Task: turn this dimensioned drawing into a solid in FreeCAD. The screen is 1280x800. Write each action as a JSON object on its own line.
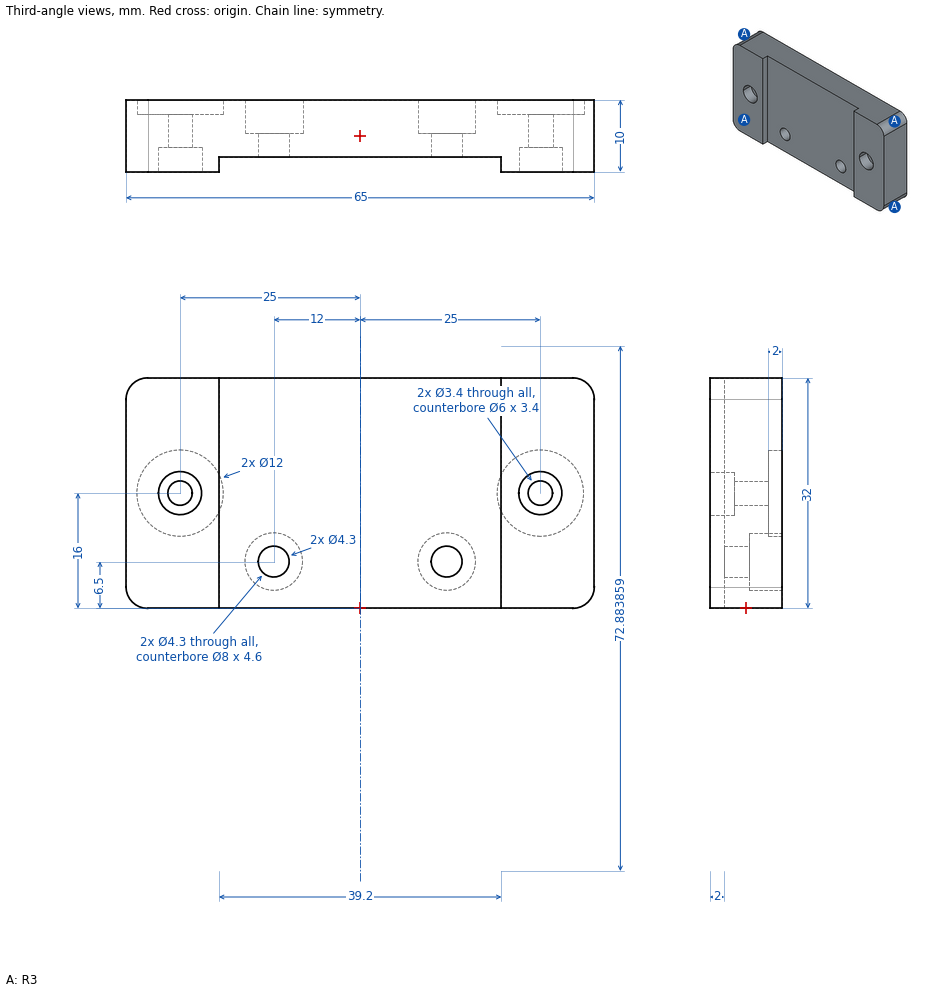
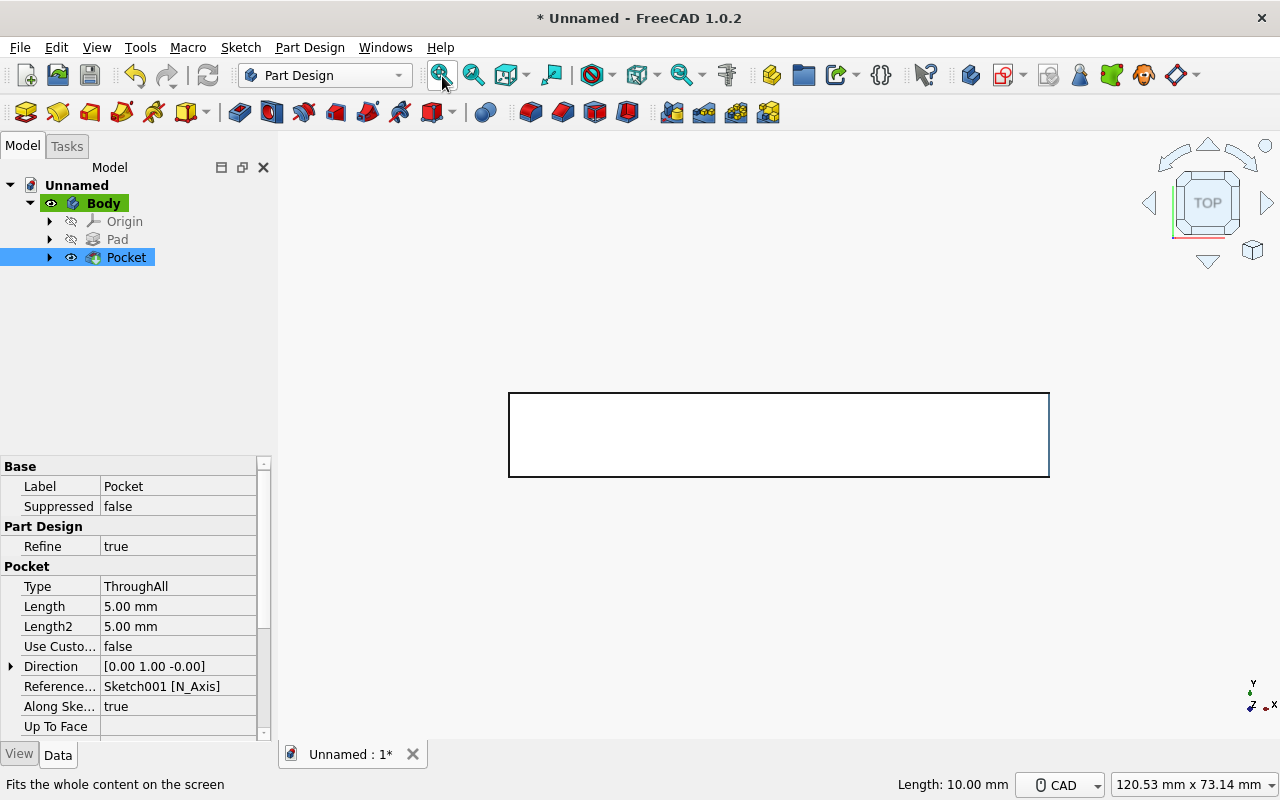
{"action": "left_click", "coordinate": [509, 434], "text": "ctrl"}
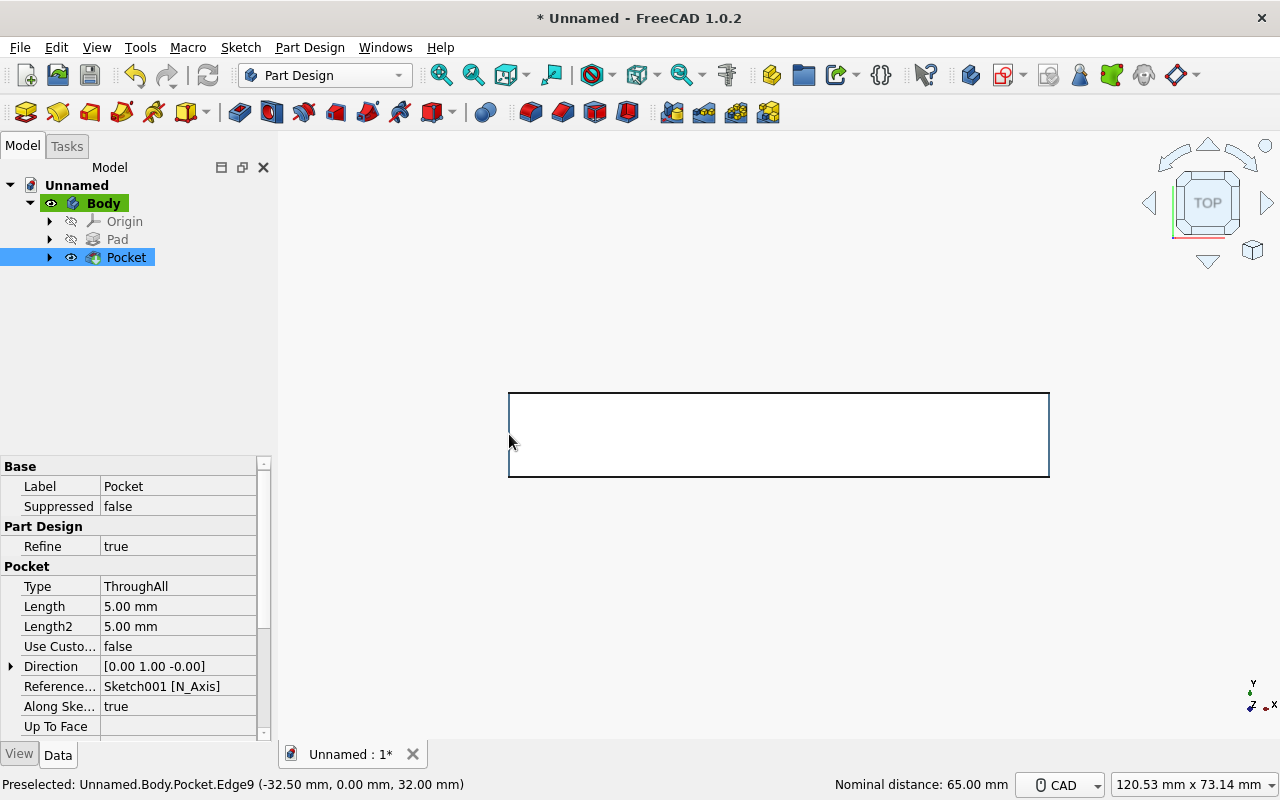
{"action": "key", "text": "1"}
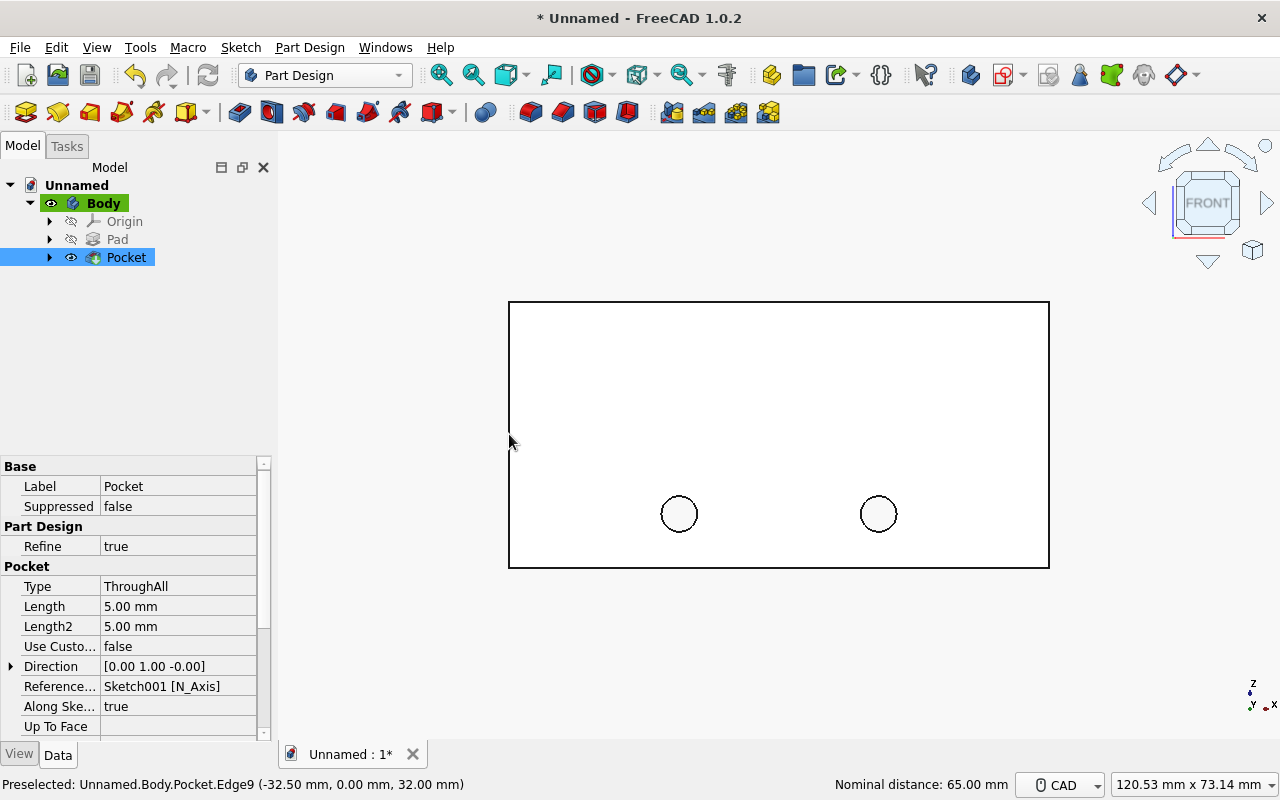
{"action": "key", "text": "3"}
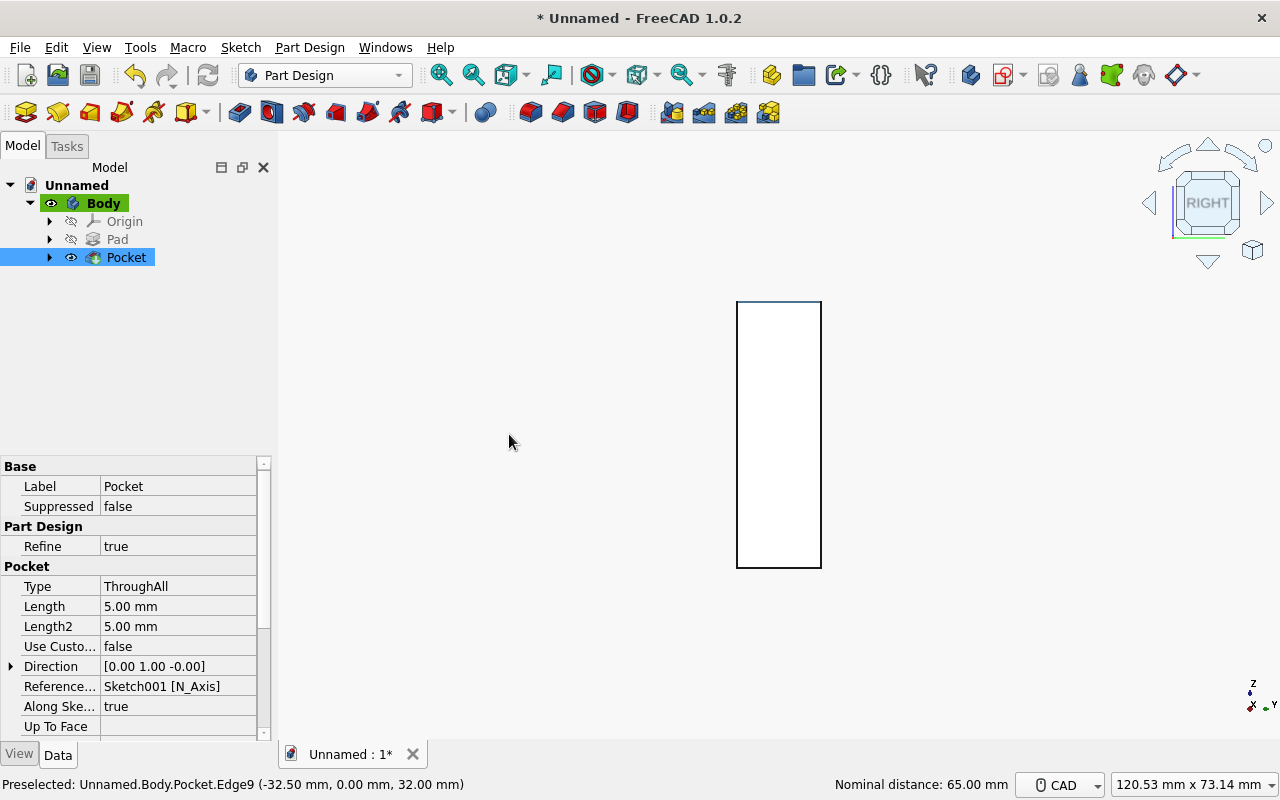
{"action": "left_click", "coordinate": [442, 76]}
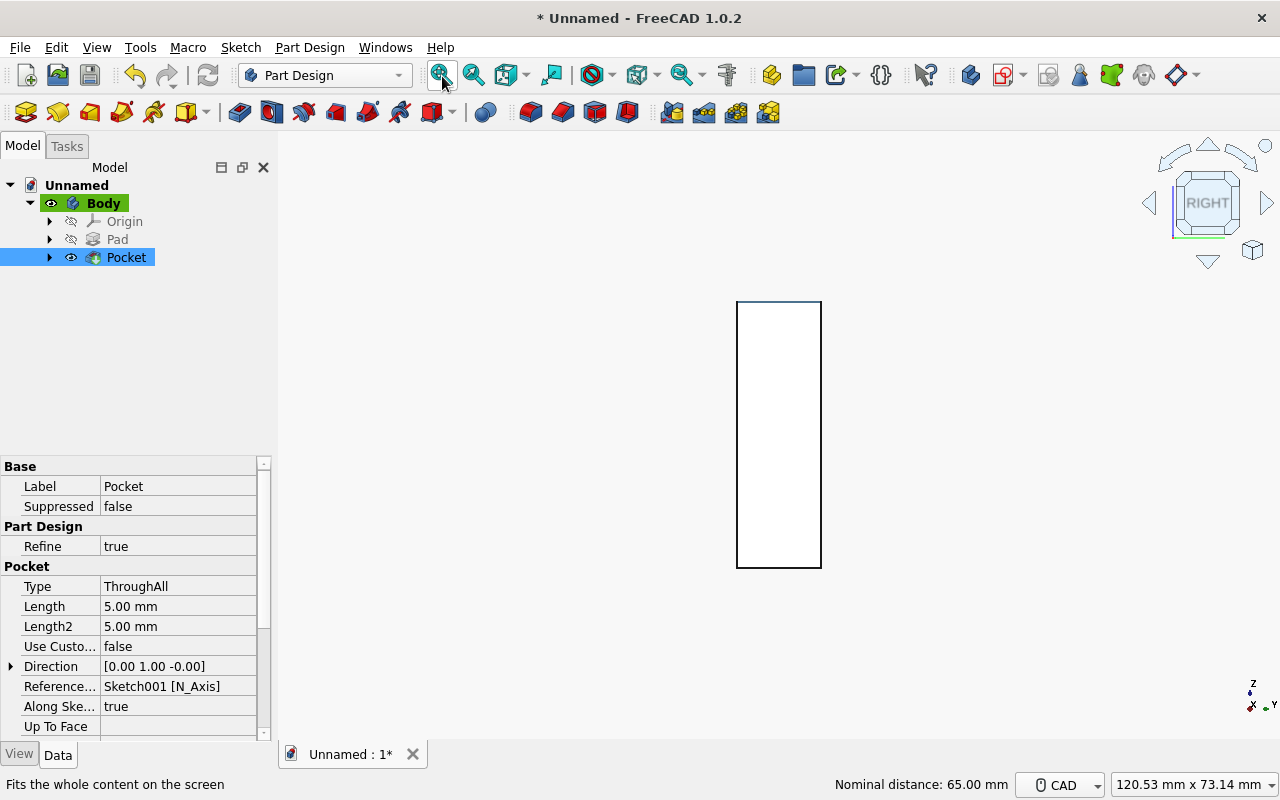
{"action": "left_click", "coordinate": [779, 567], "text": "ctrl"}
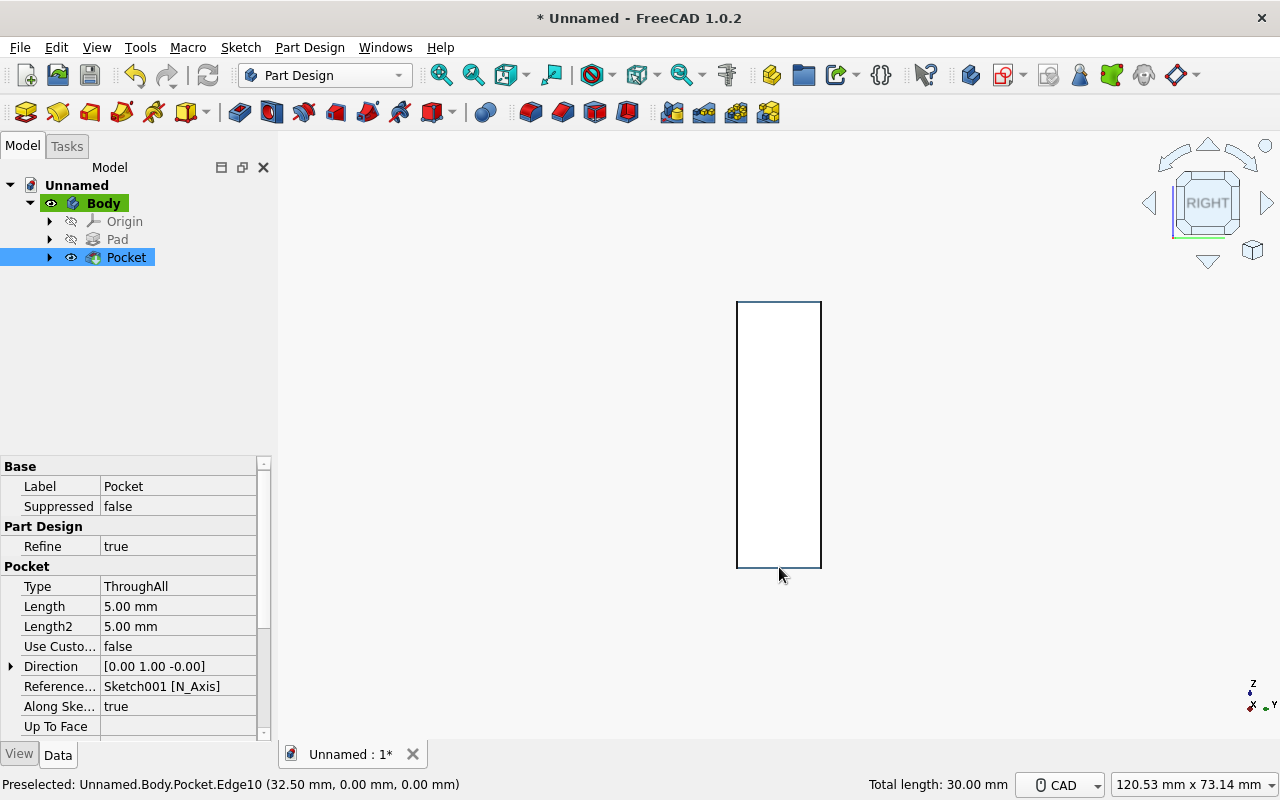
{"action": "key", "text": "5"}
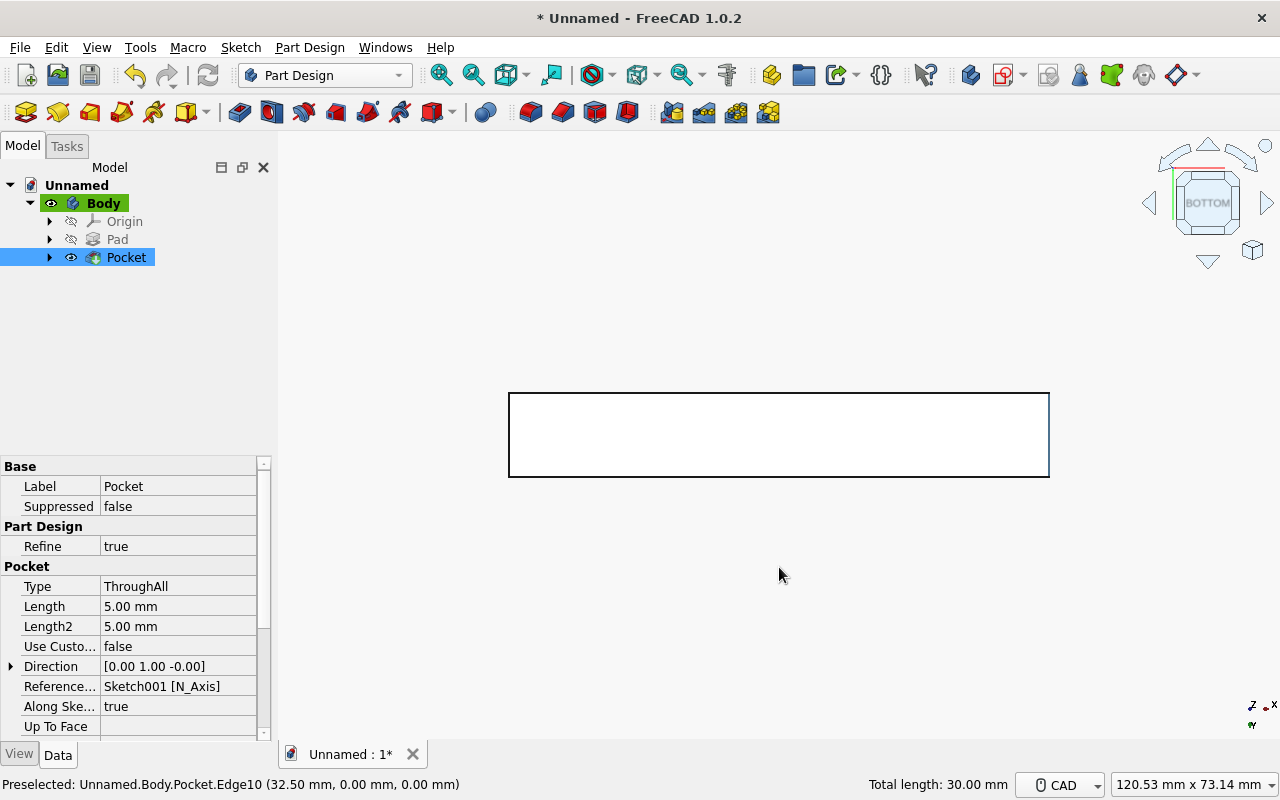
{"action": "left_click", "coordinate": [509, 434], "text": "ctrl"}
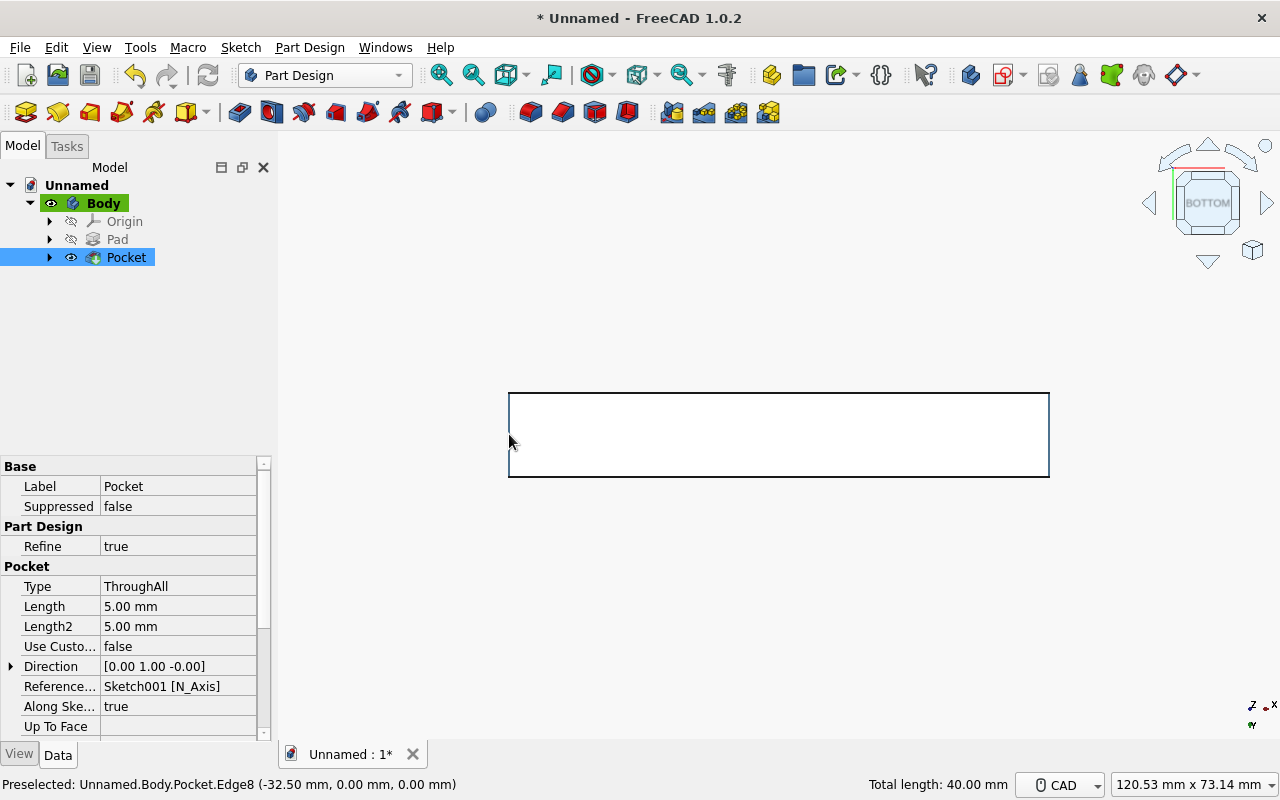
{"action": "left_click", "coordinate": [532, 112]}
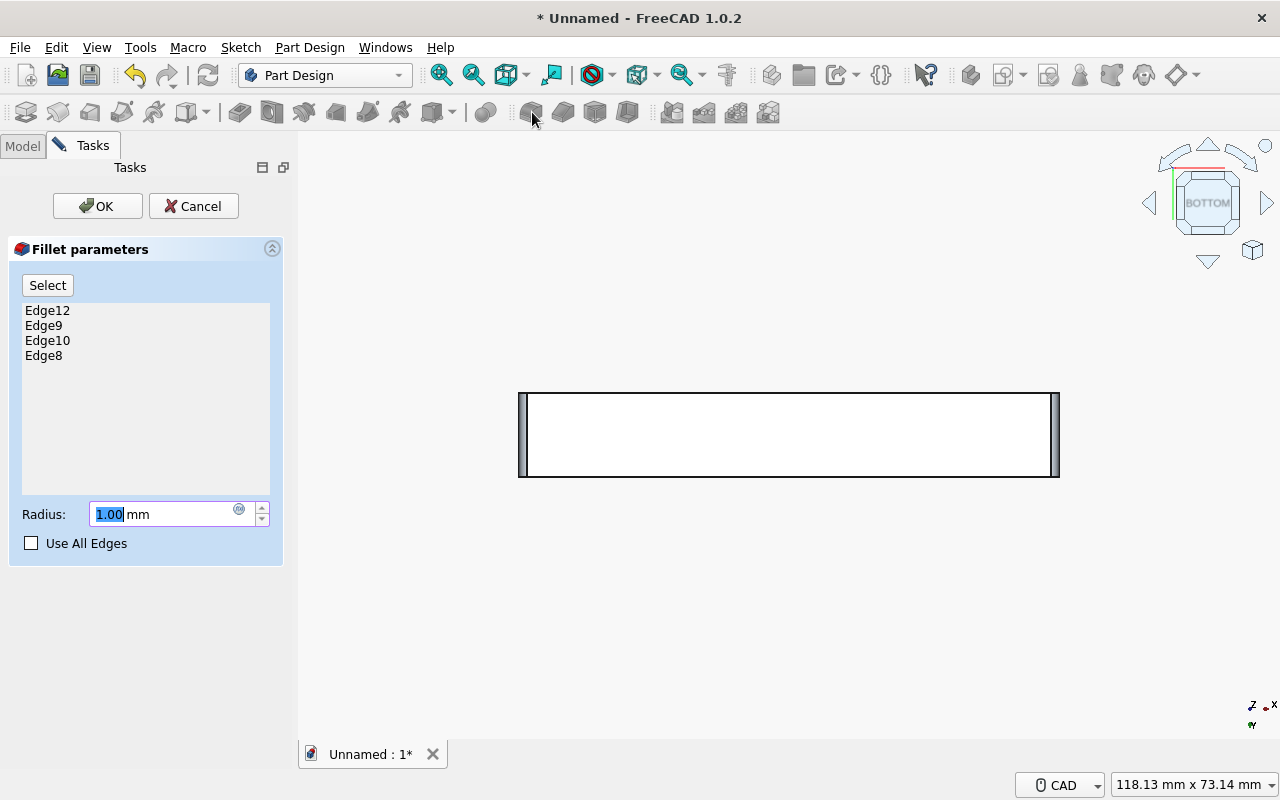
{"action": "type", "text": "3"}
{"action": "key", "text": "Tab"}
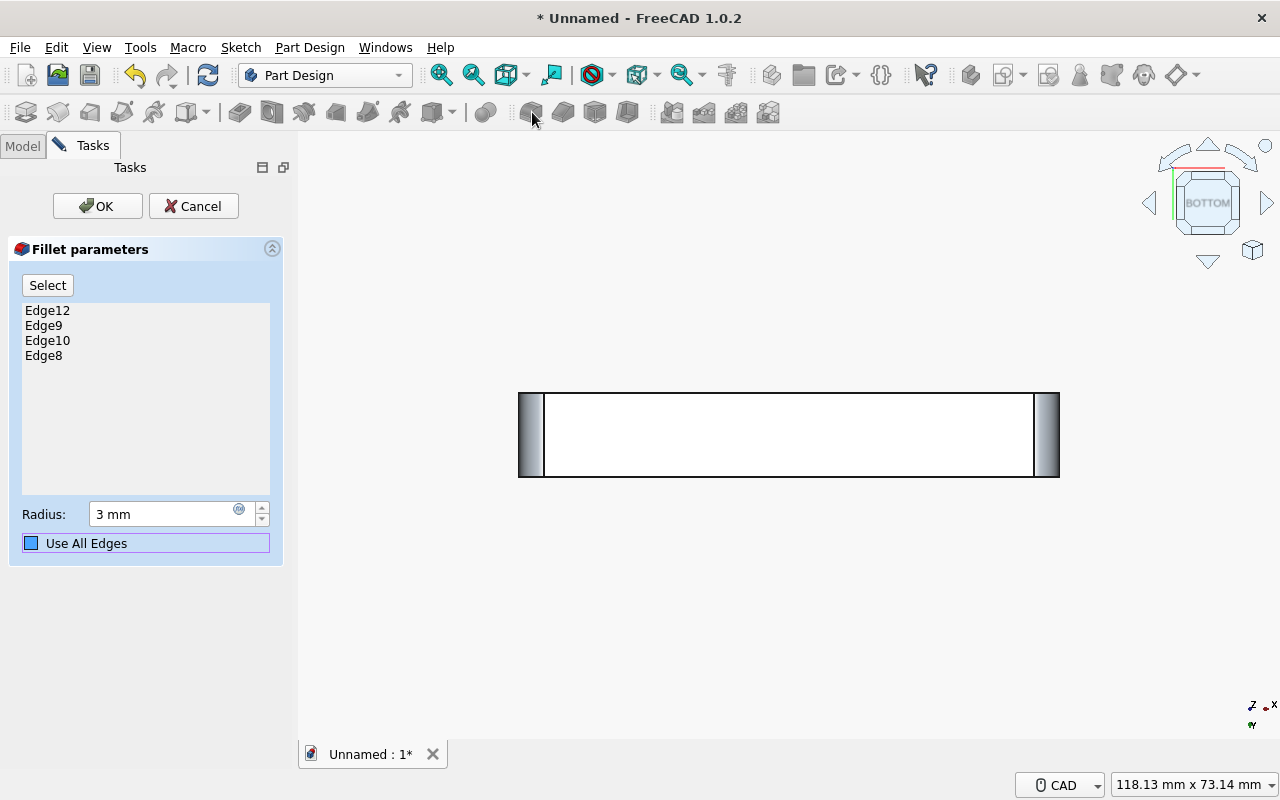
{"action": "left_click", "coordinate": [98, 206]}